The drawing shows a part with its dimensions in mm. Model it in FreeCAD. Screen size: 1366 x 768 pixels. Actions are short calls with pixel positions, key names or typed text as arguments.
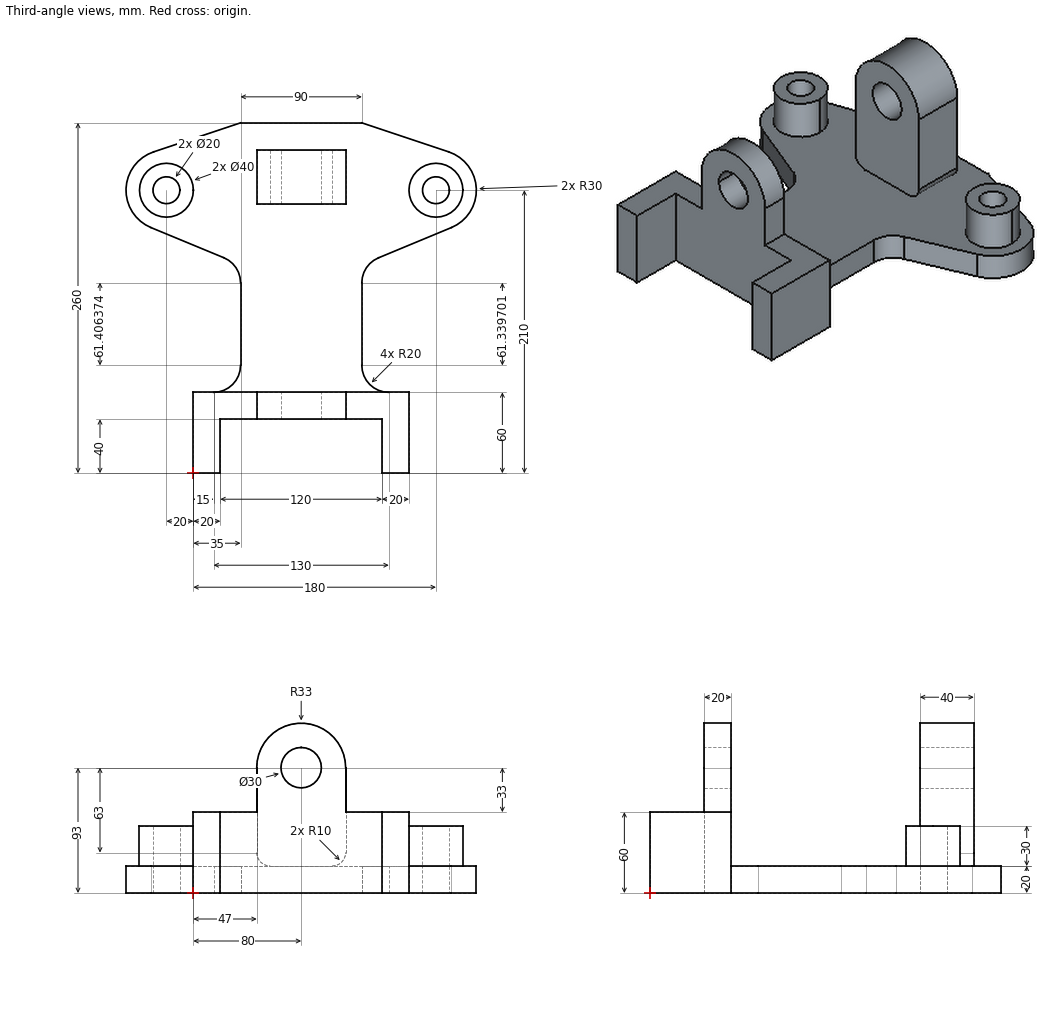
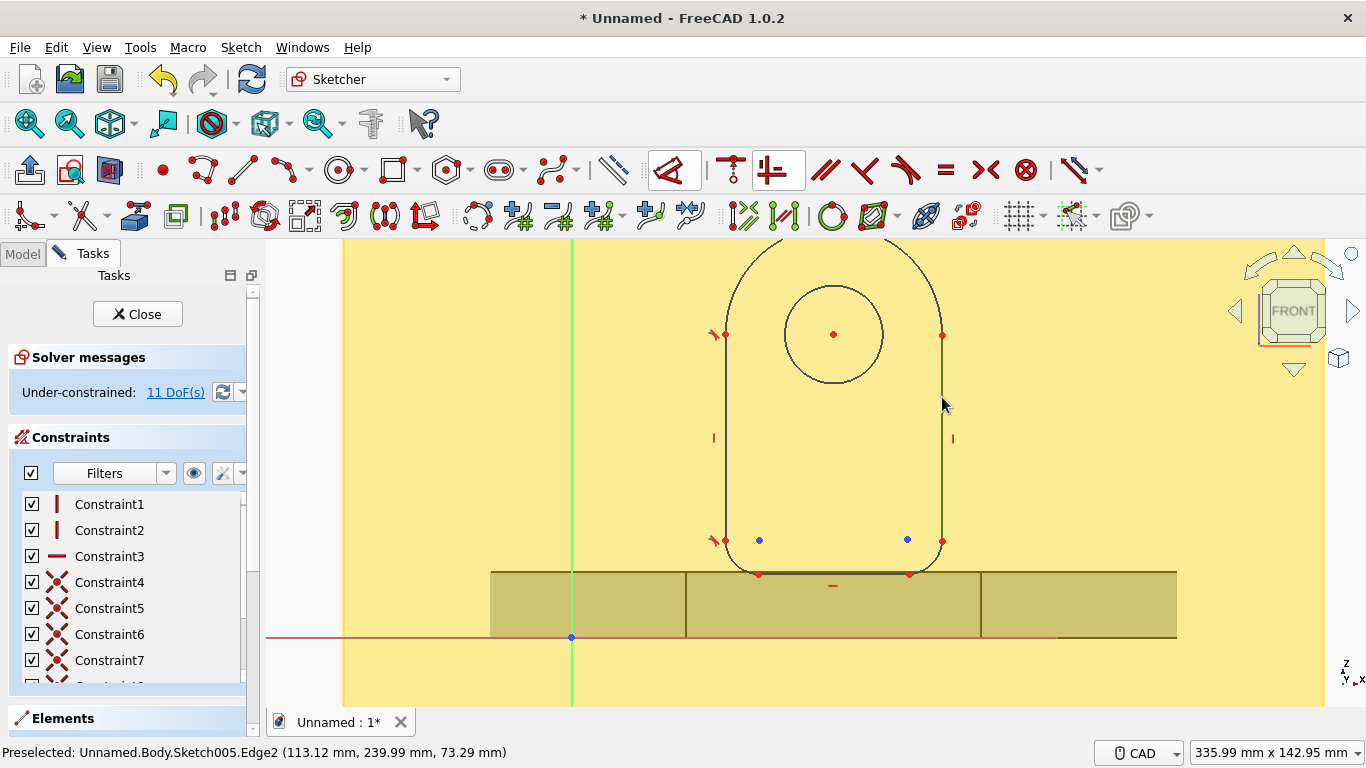
click(922, 271)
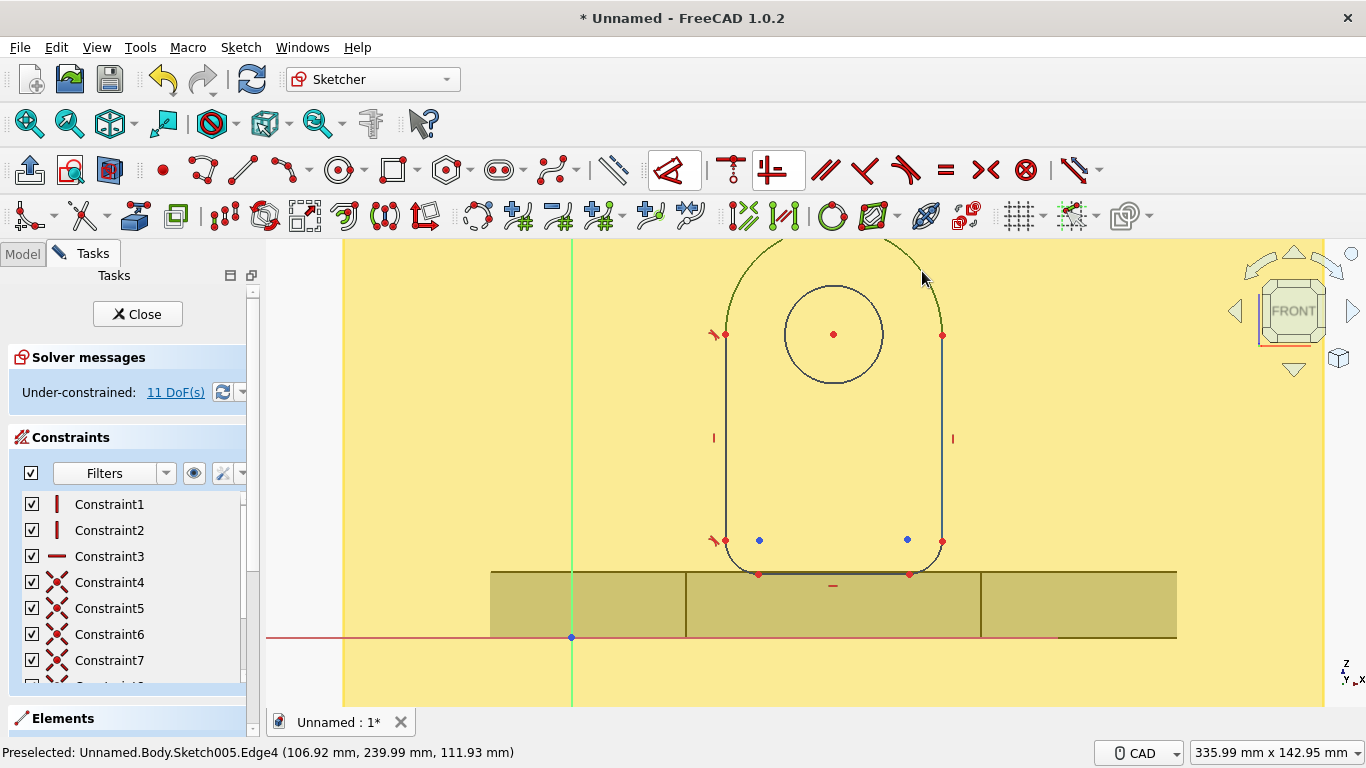
click(906, 170)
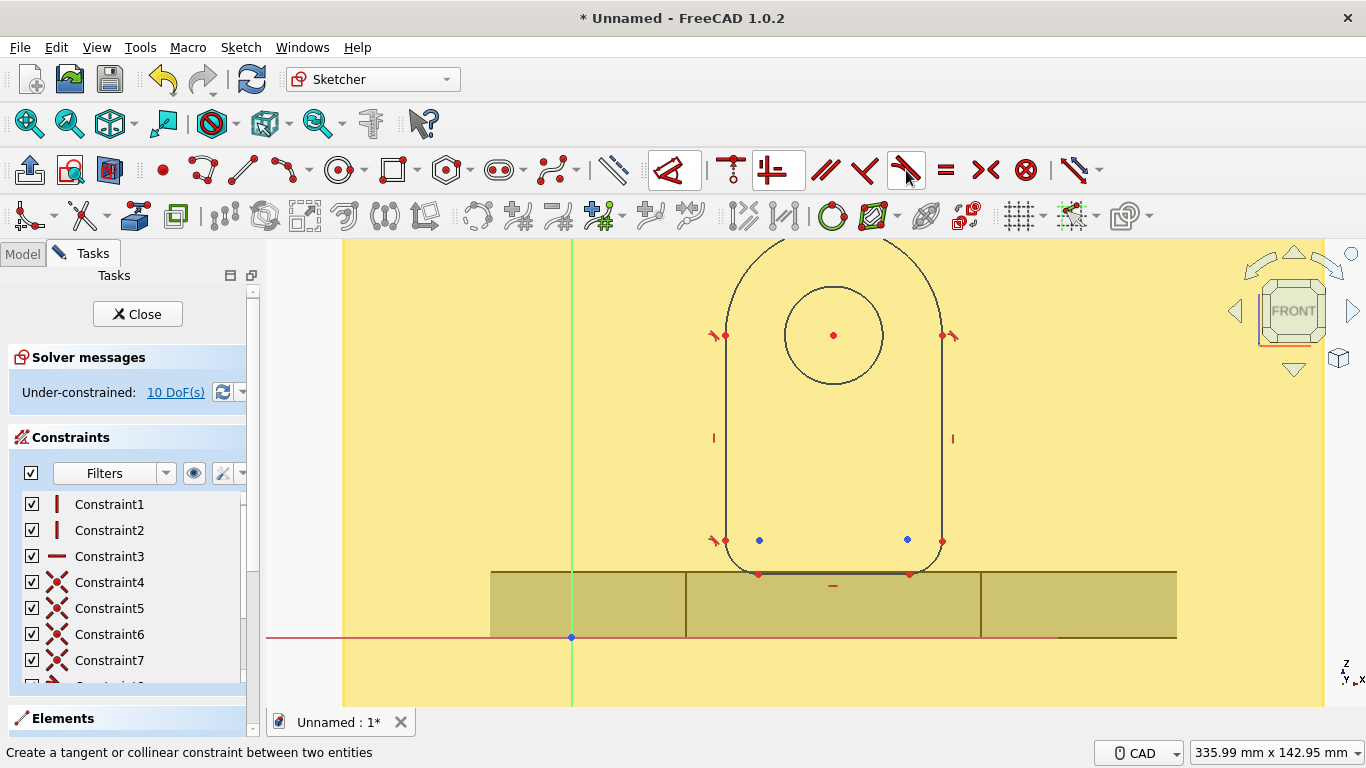
click(942, 397)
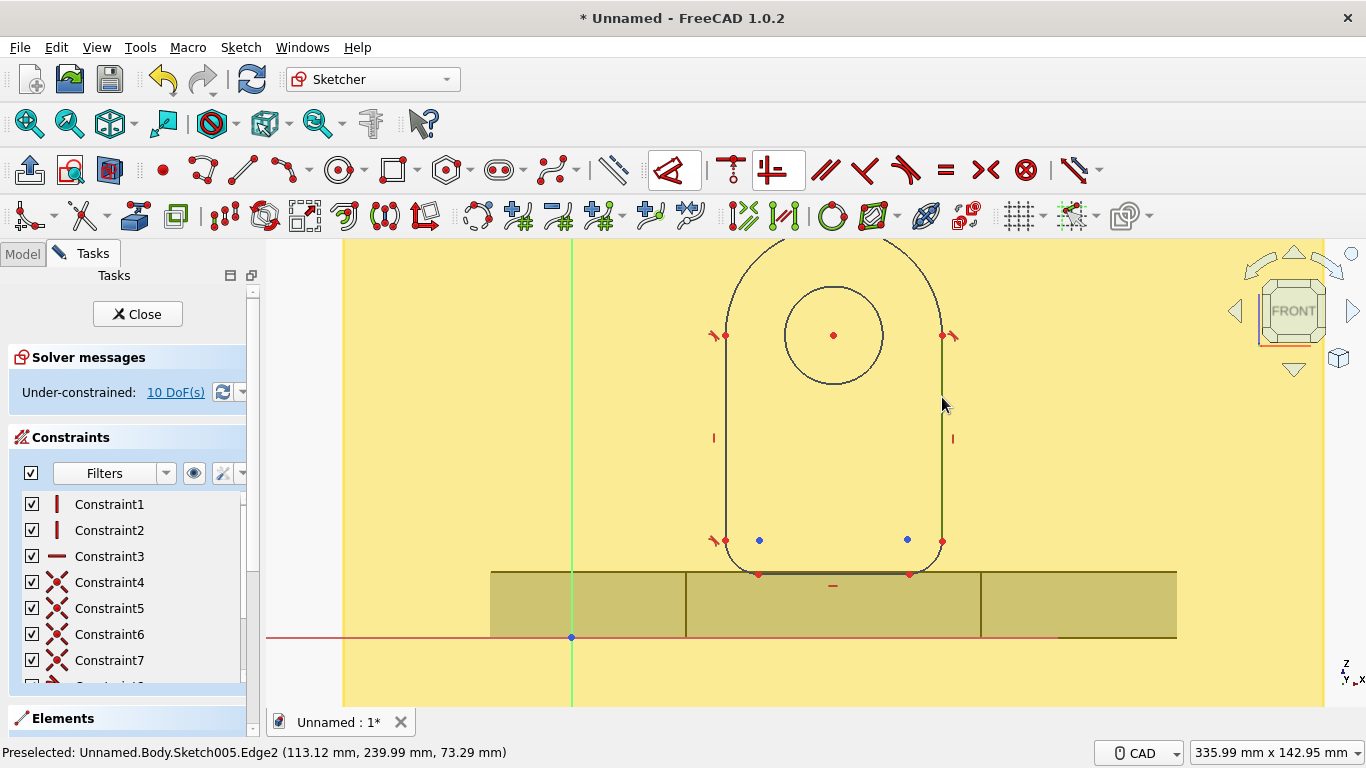
click(924, 570)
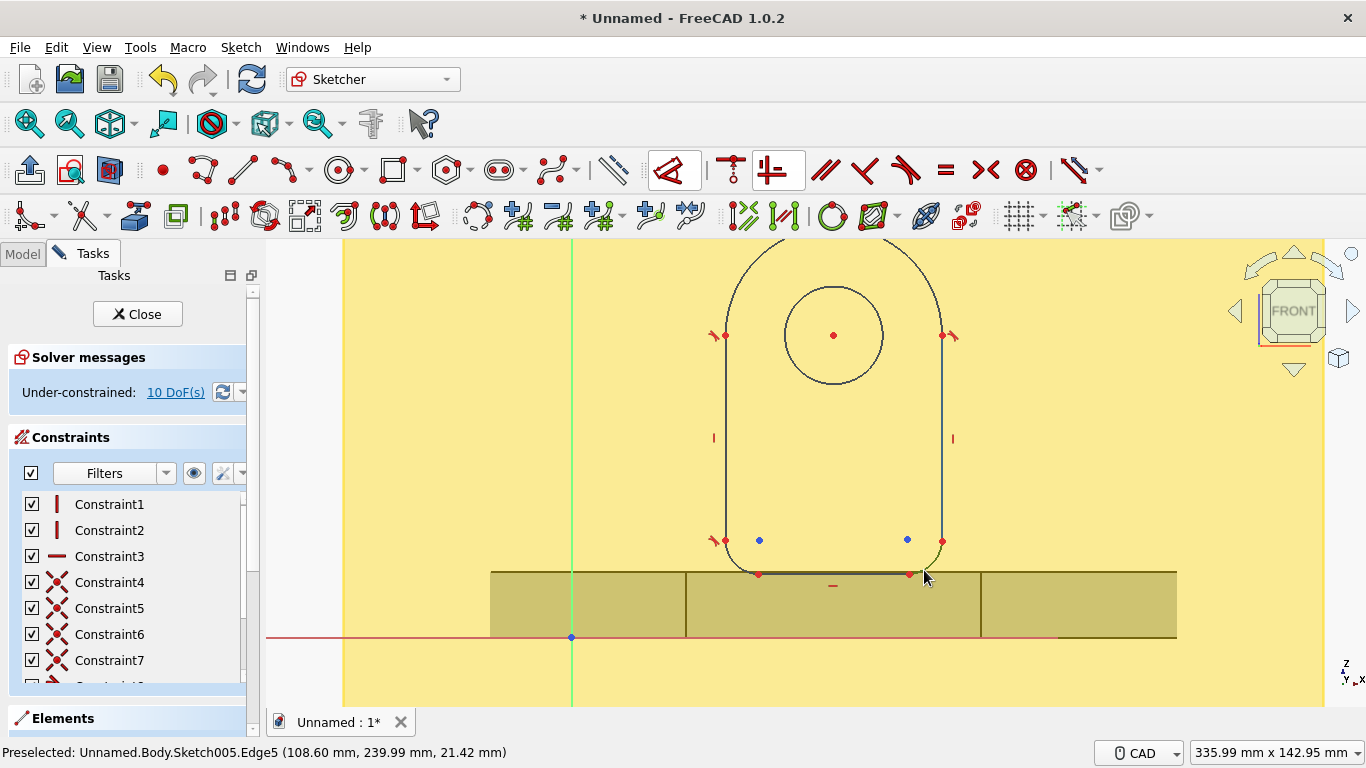
key(t)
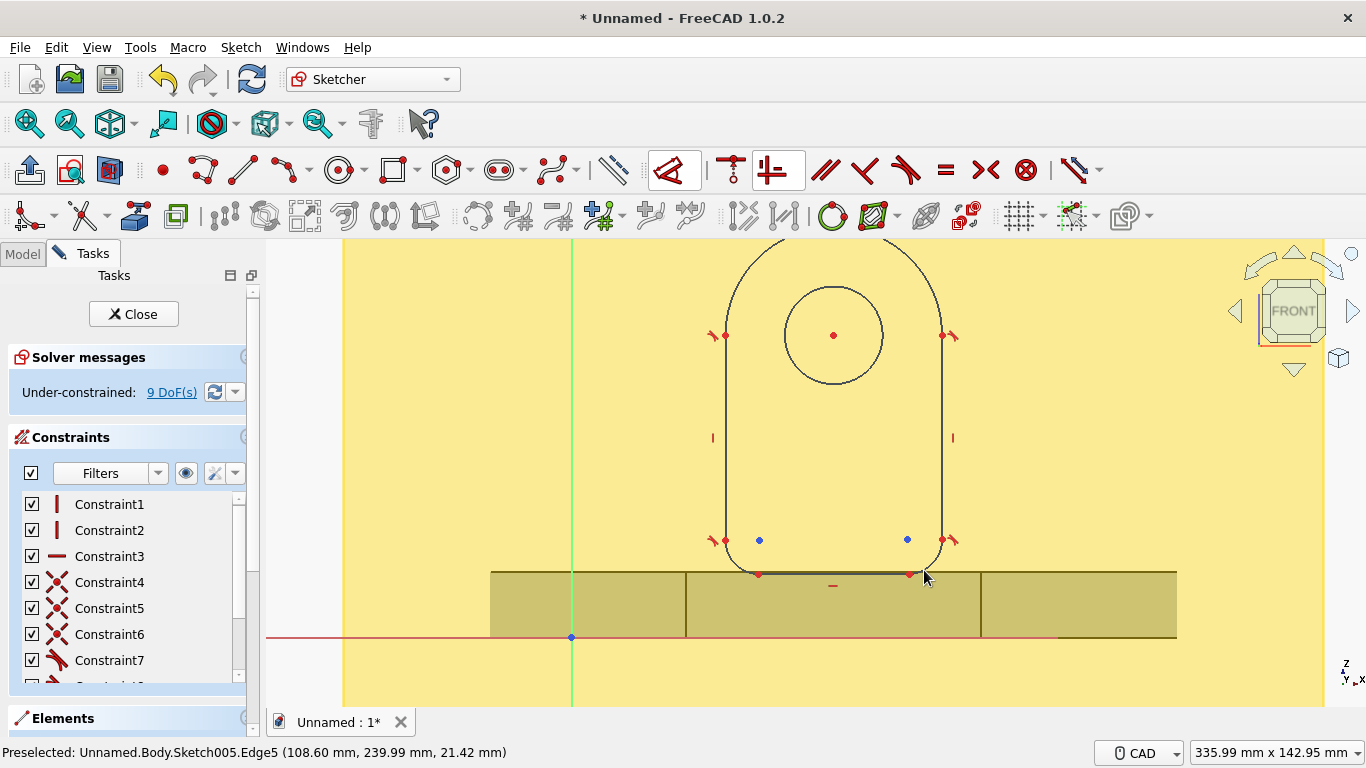
click(864, 574)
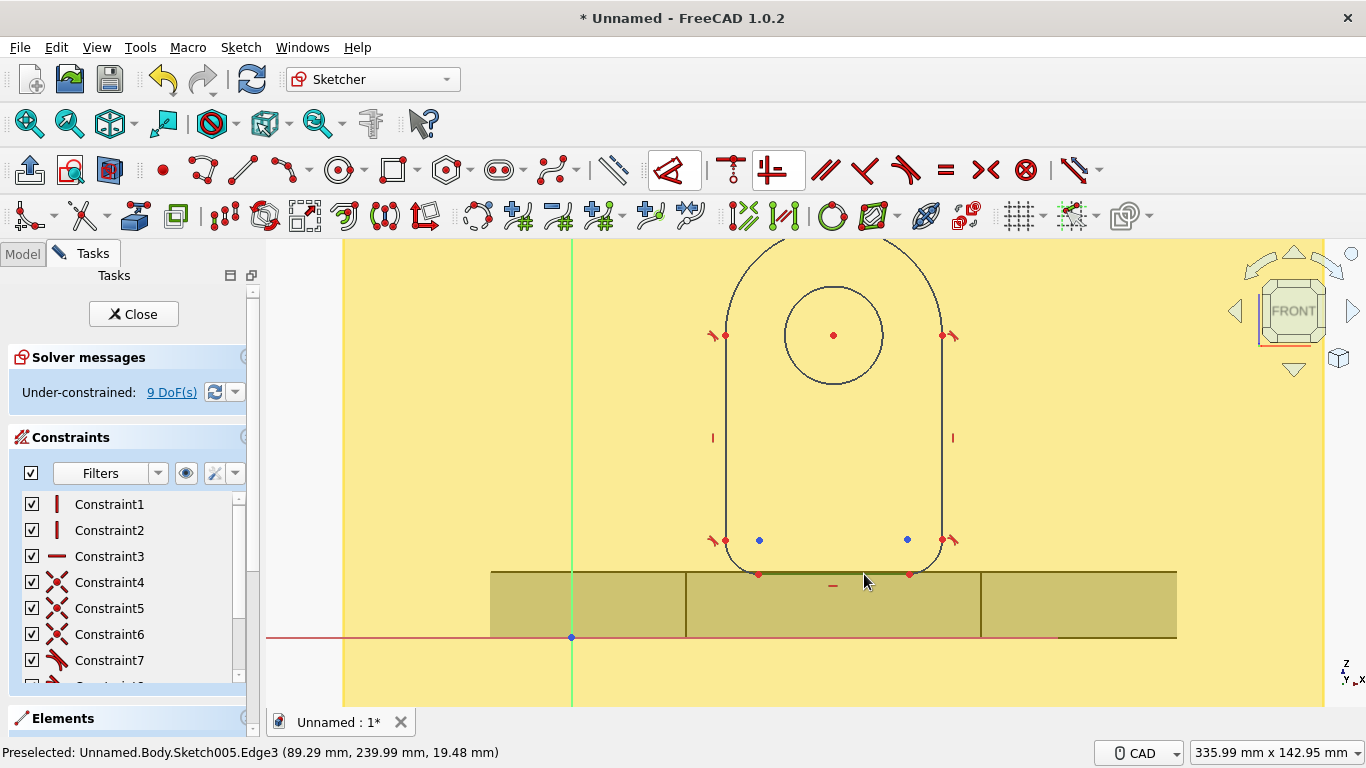
click(924, 570)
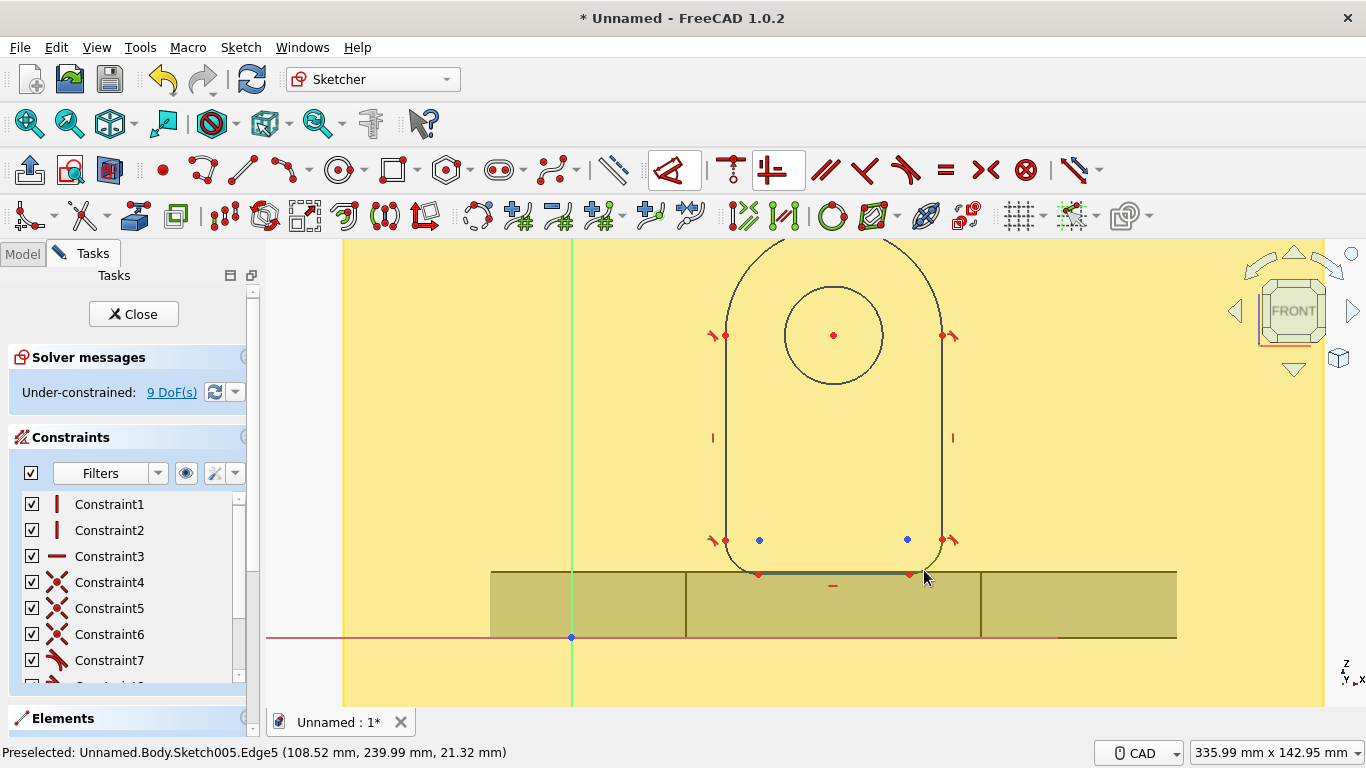
click(906, 170)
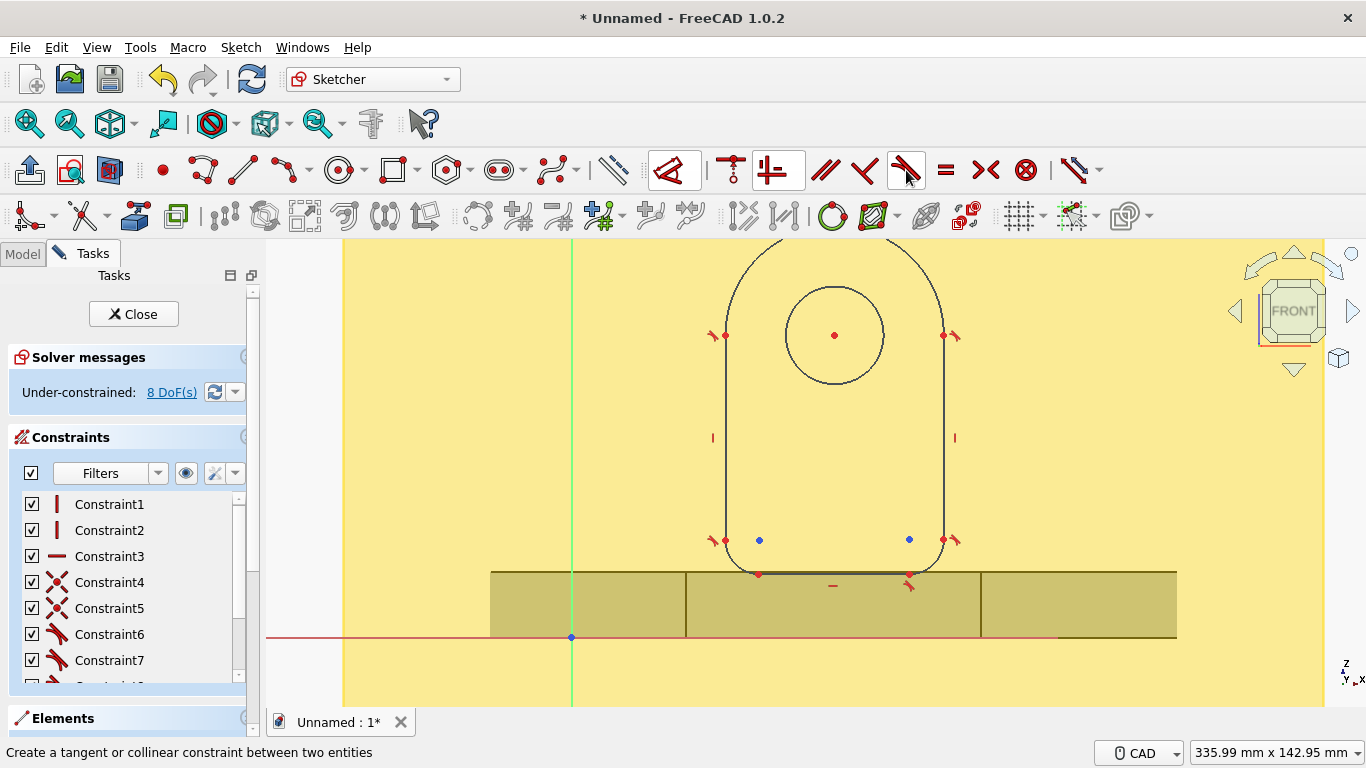
click(864, 574)